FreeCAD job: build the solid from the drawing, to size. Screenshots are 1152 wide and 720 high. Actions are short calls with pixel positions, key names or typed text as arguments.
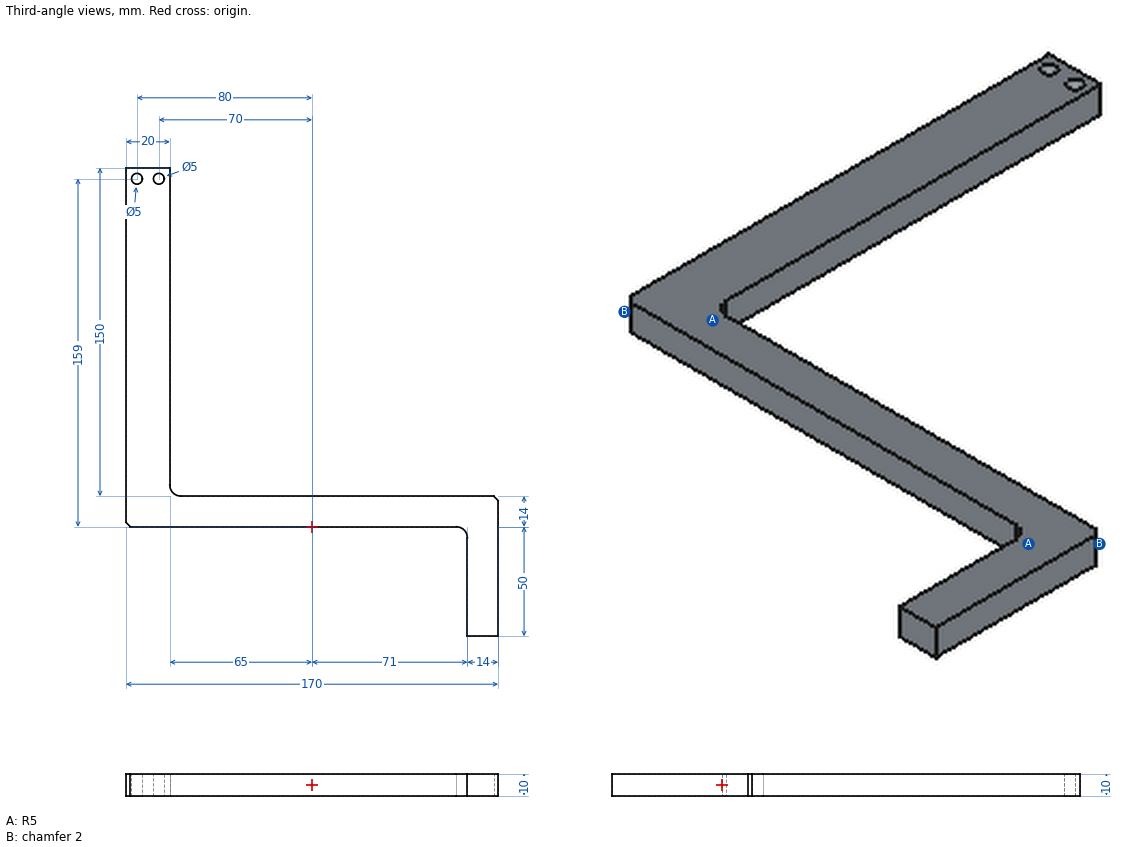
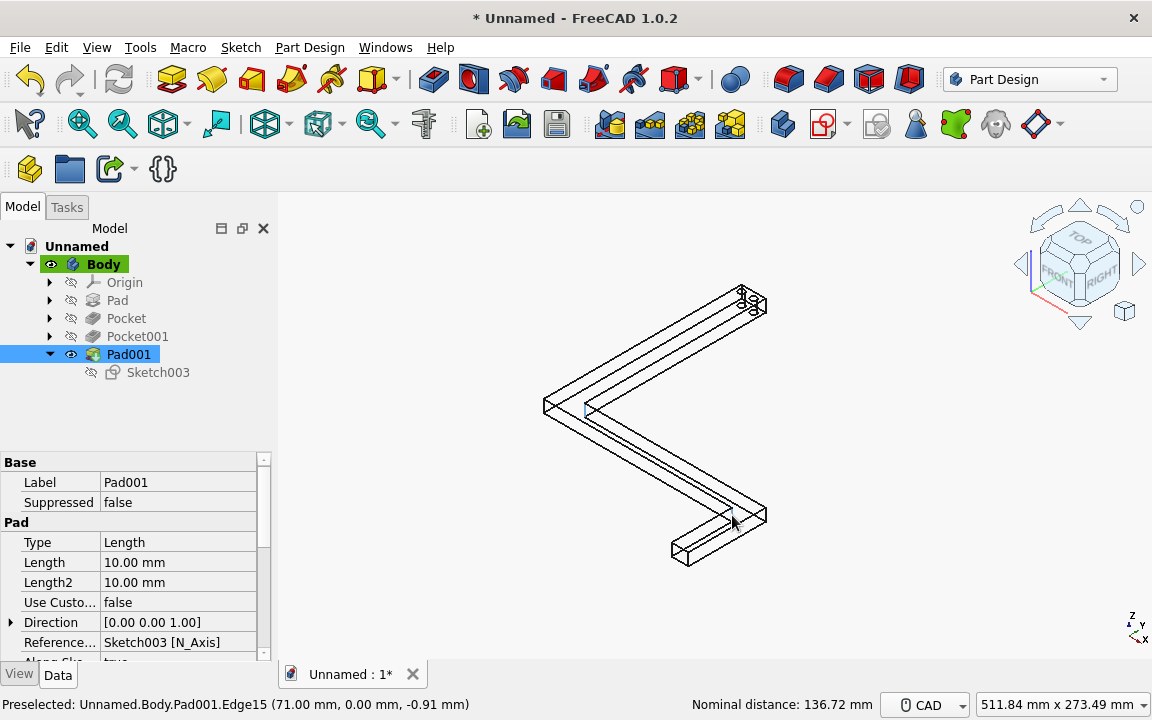
key(v)
key(1)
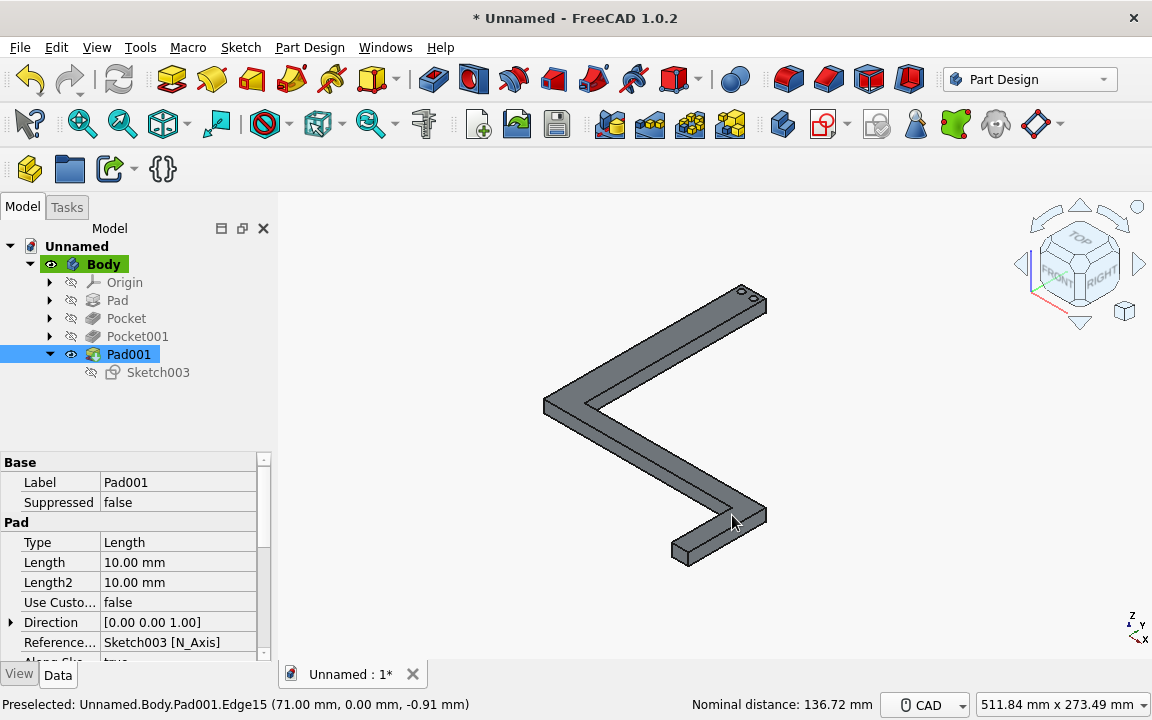
click(790, 80)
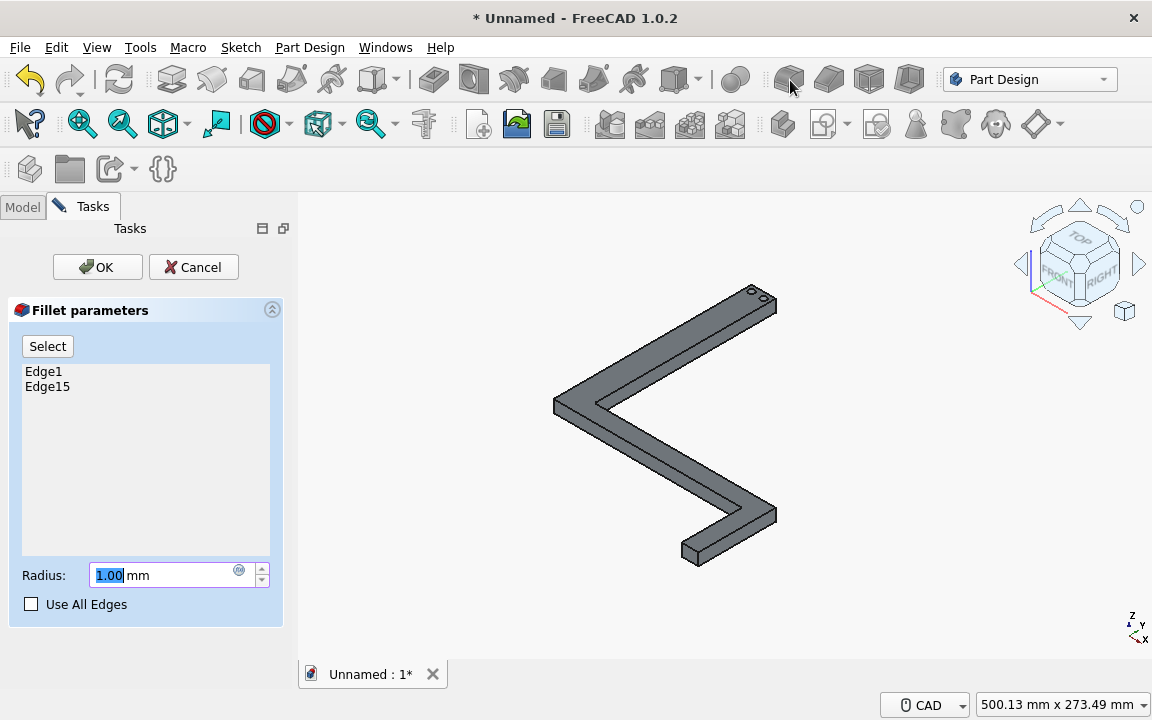
text(5)
key(Tab)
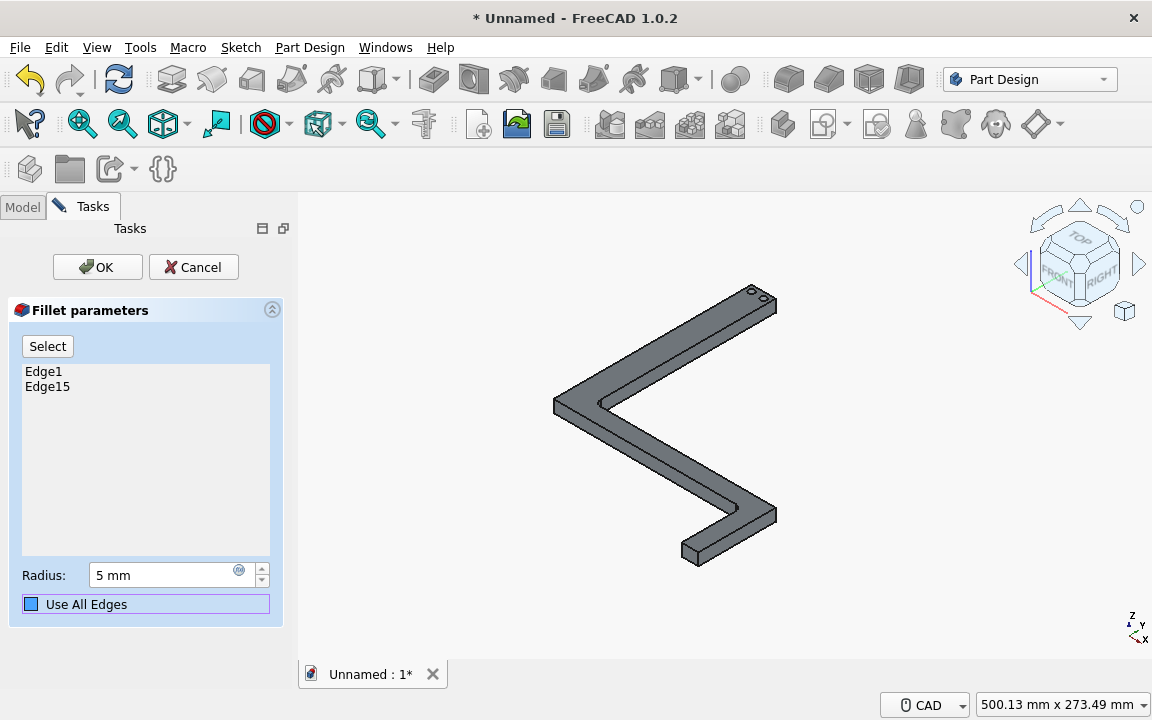
click(98, 267)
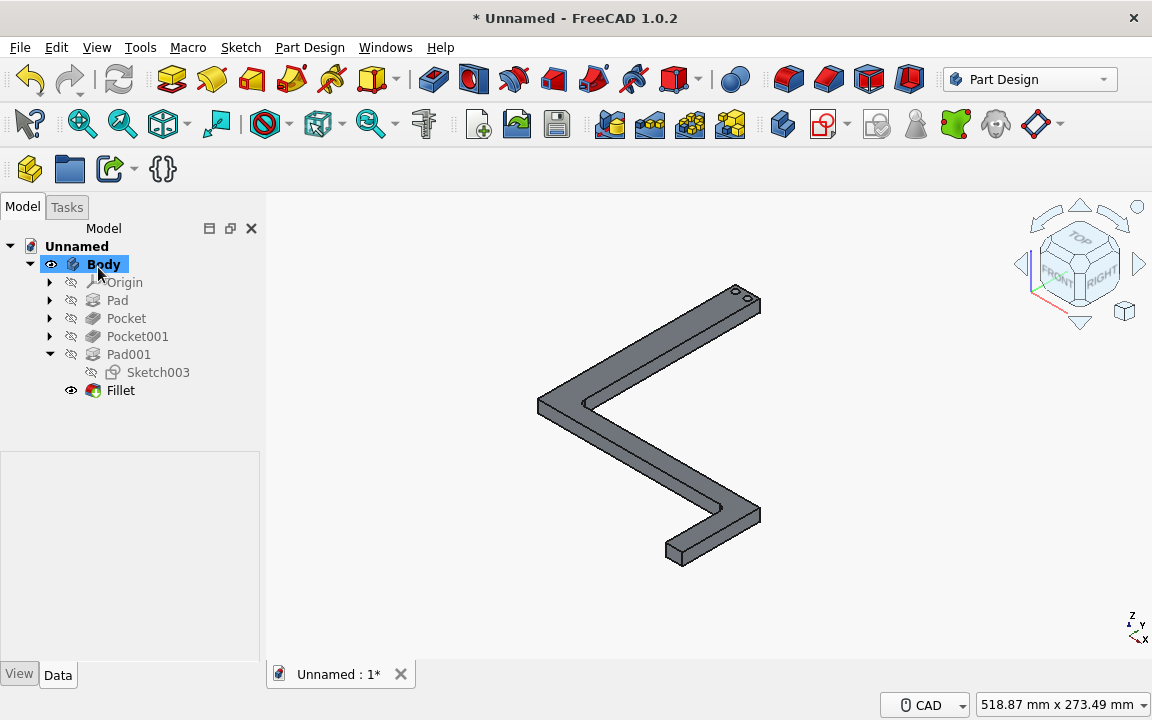
scroll(538, 405, up, 5)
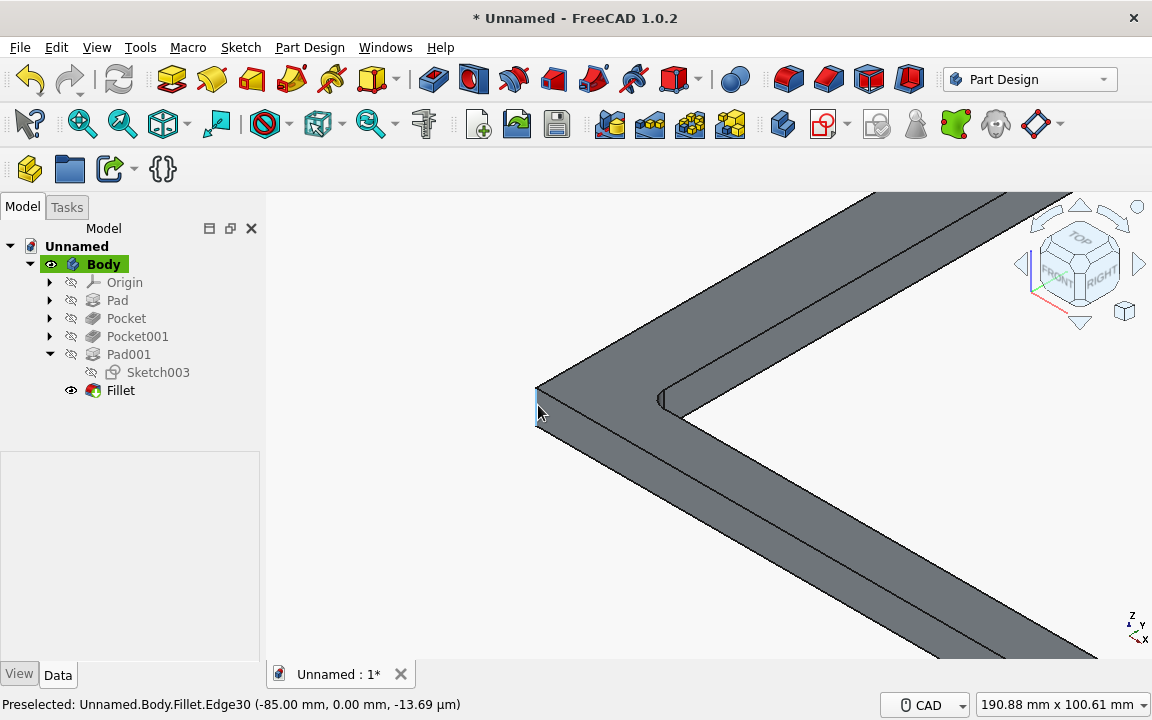
key(v)
key(f)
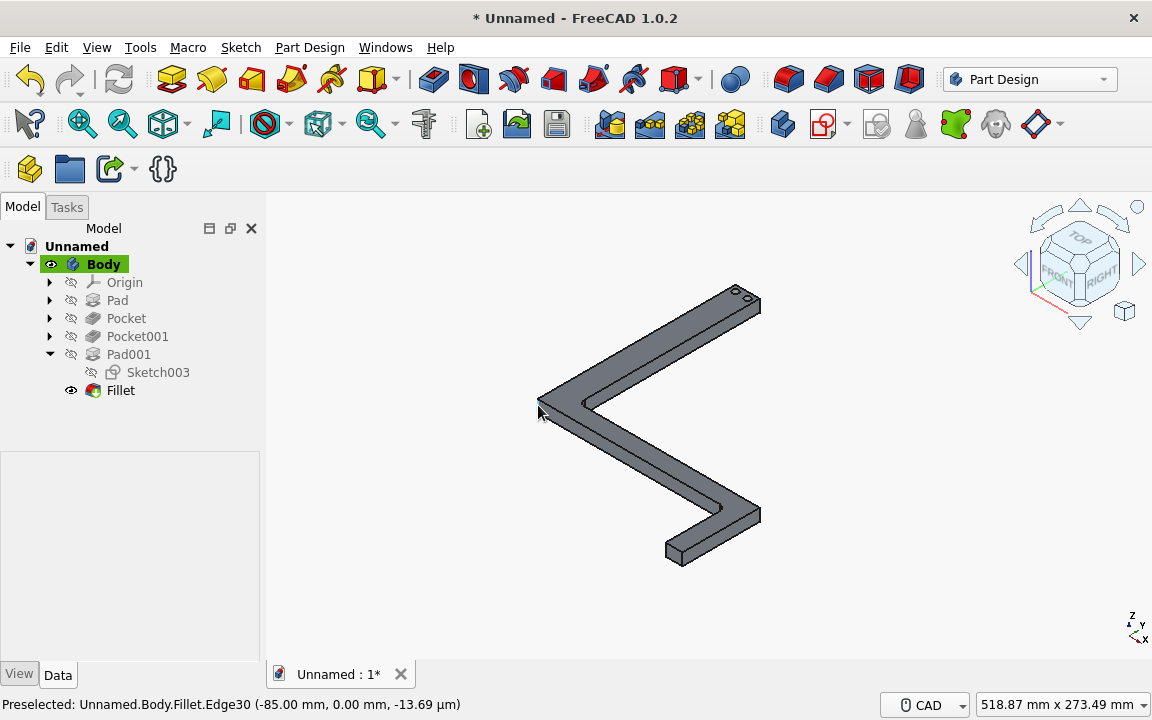
key(2)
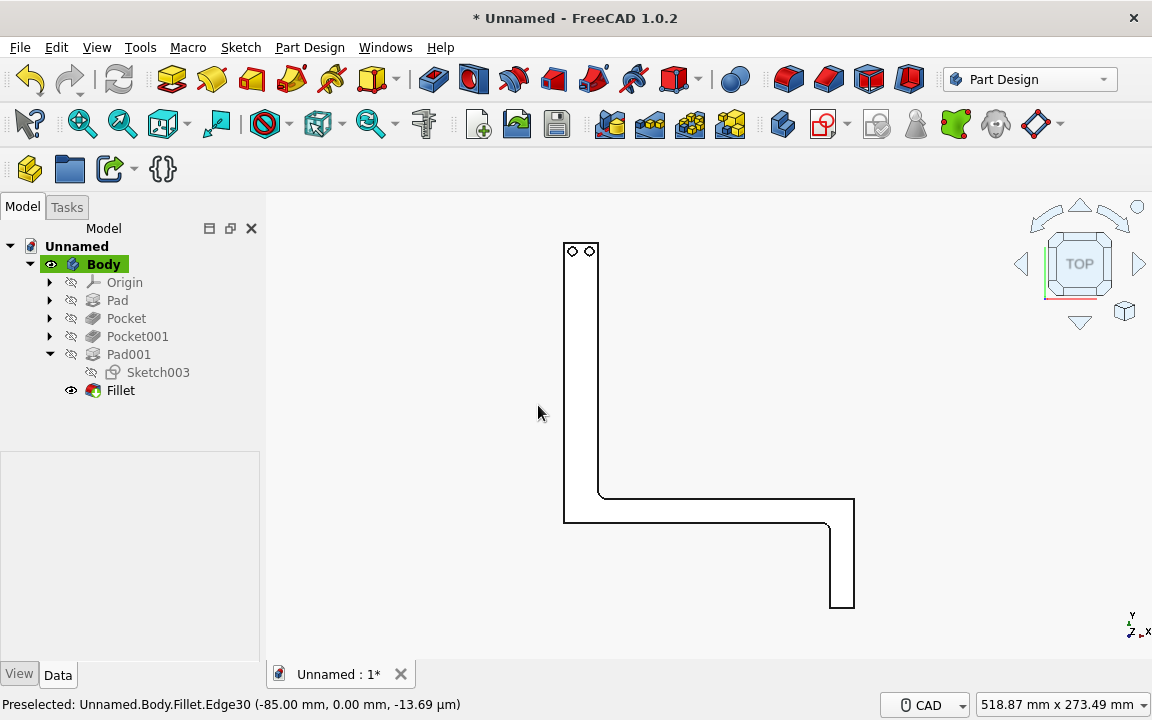
scroll(564, 522, up, 5)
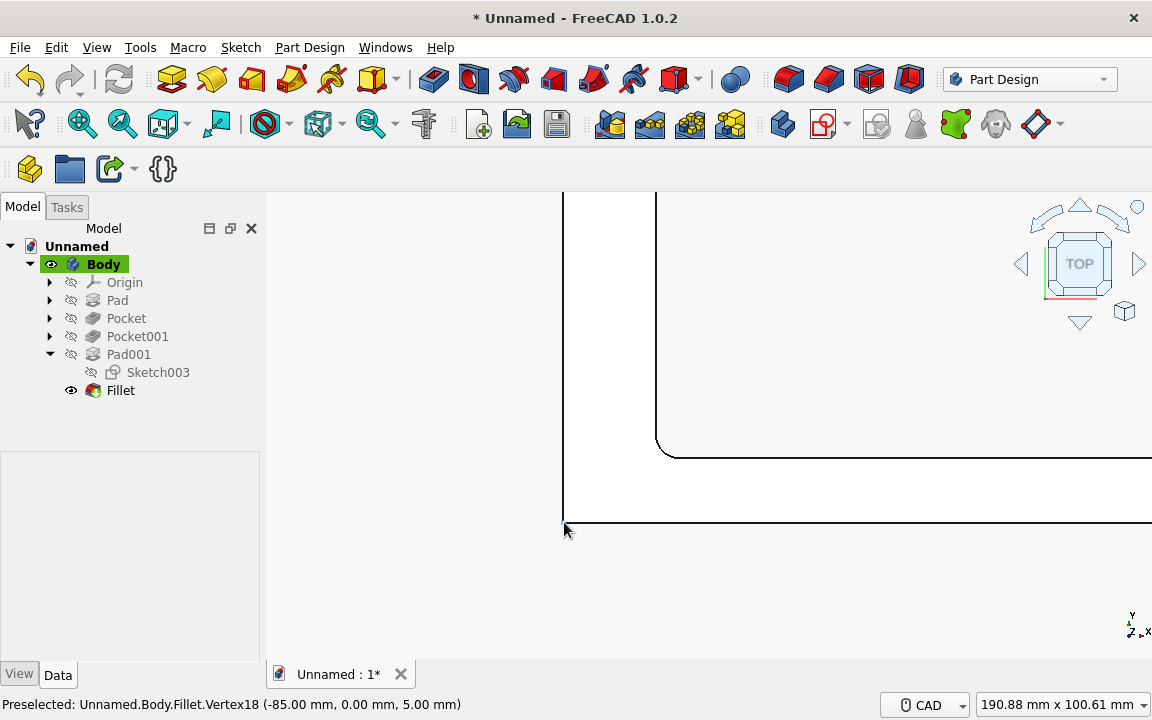
click(84, 124)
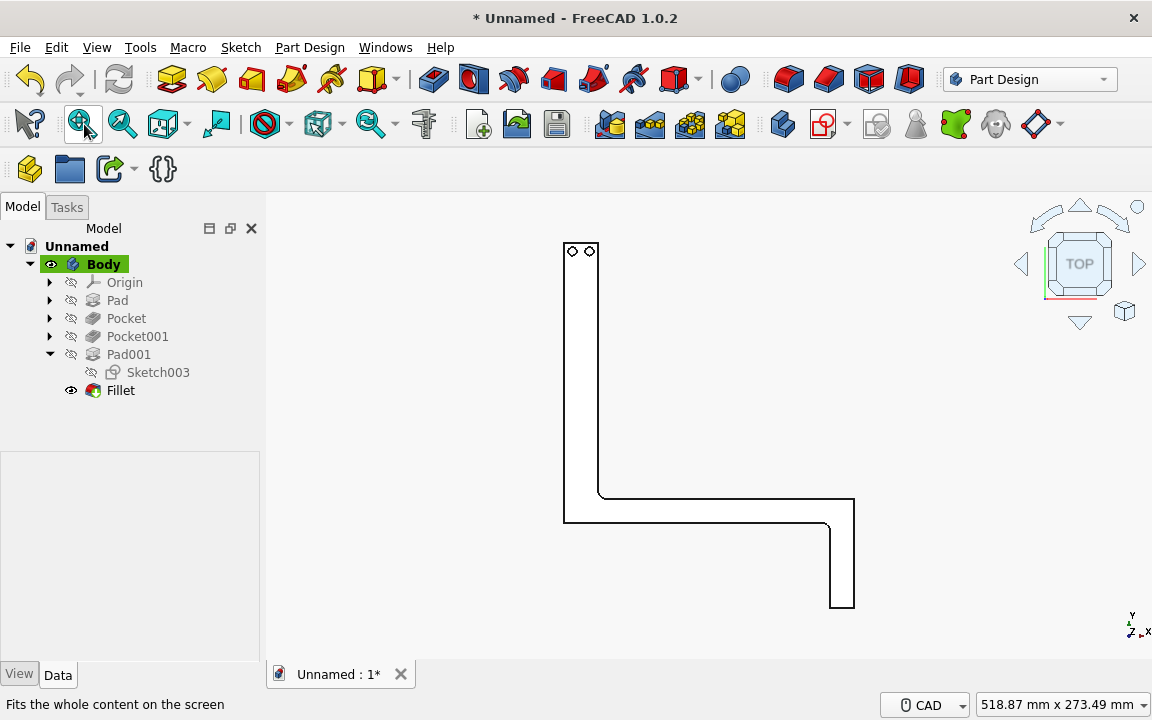
key(0)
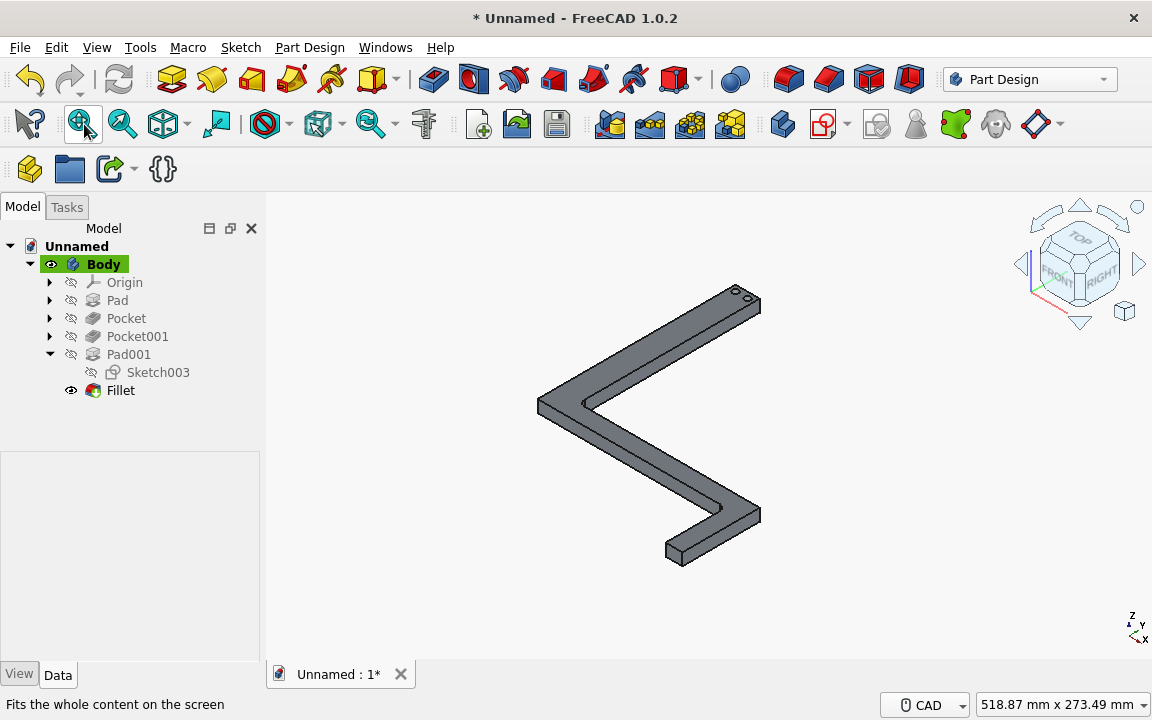
scroll(538, 405, up, 5)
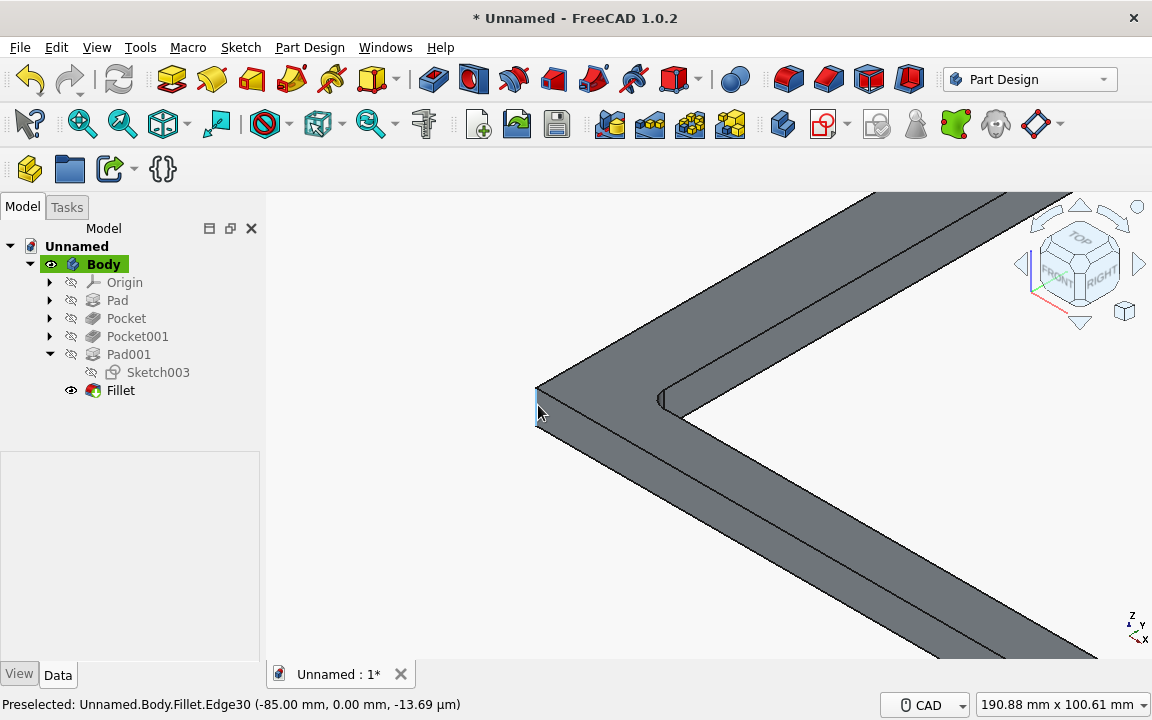
click(84, 124)